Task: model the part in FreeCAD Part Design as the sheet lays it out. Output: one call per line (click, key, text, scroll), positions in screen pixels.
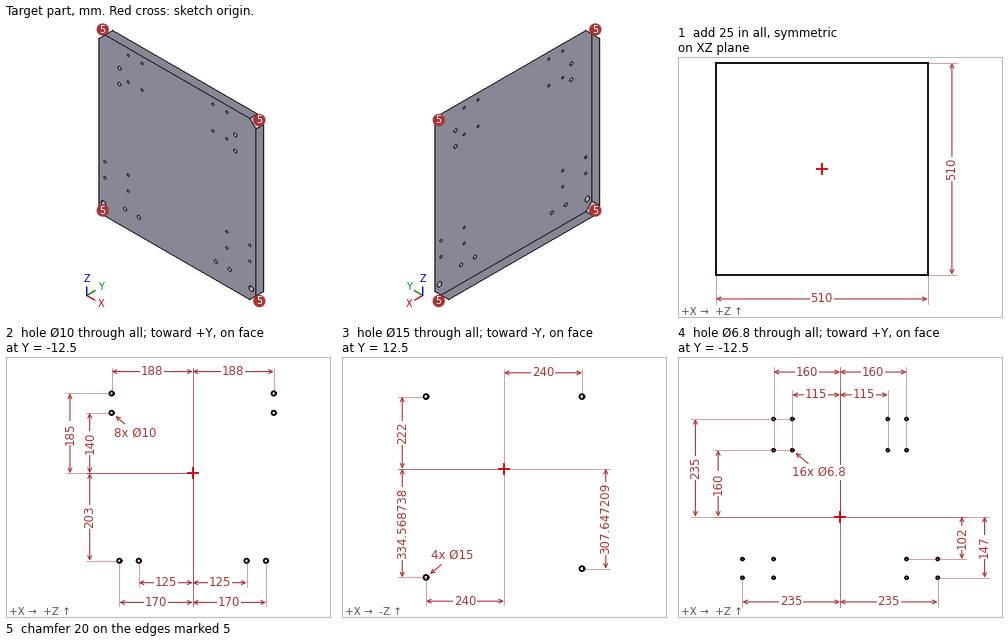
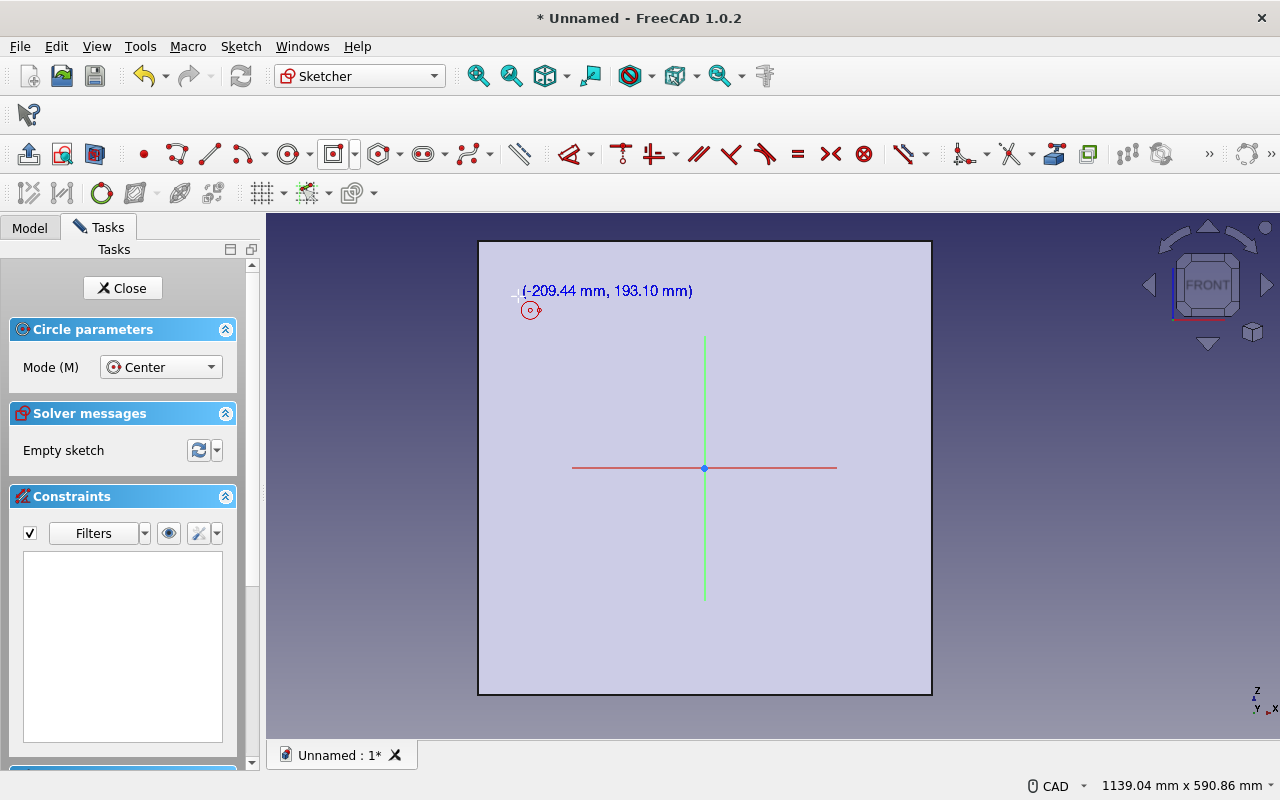
click(537, 304)
move(540, 300)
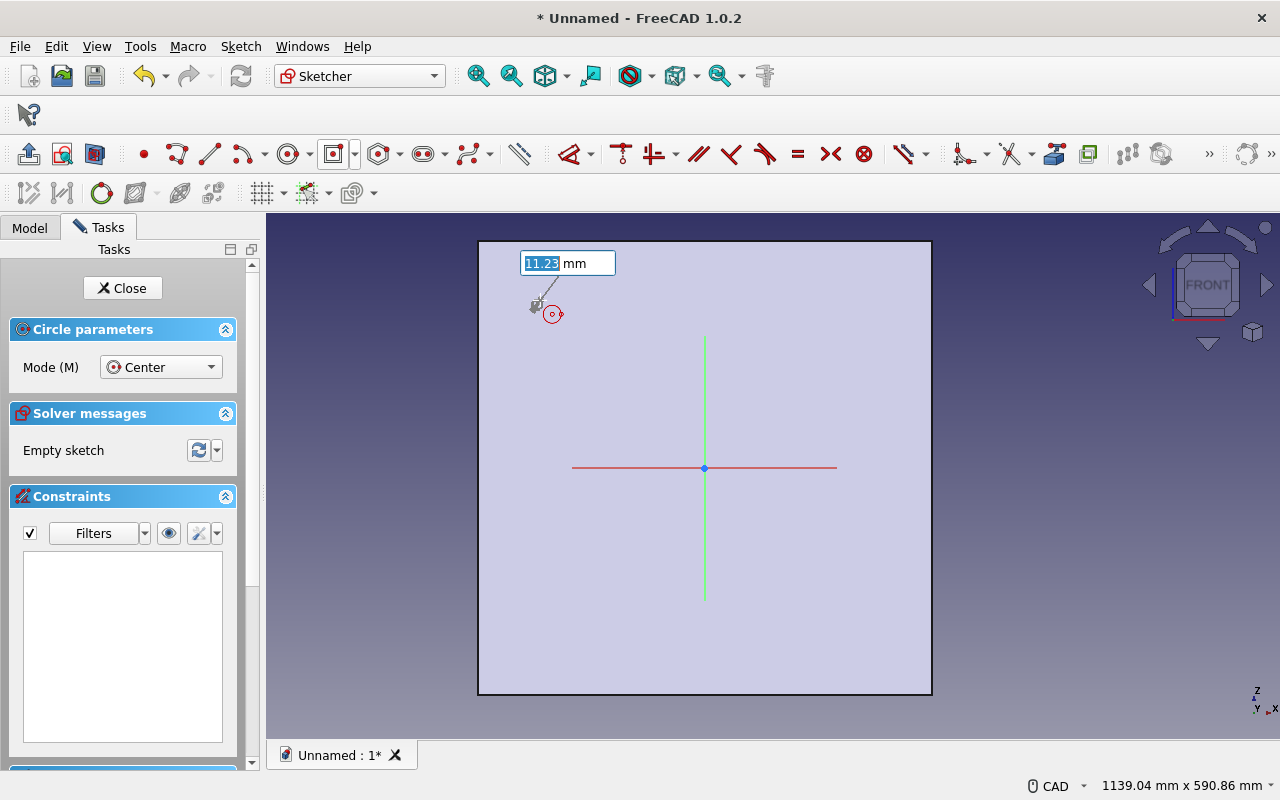
text(10)
key(Return)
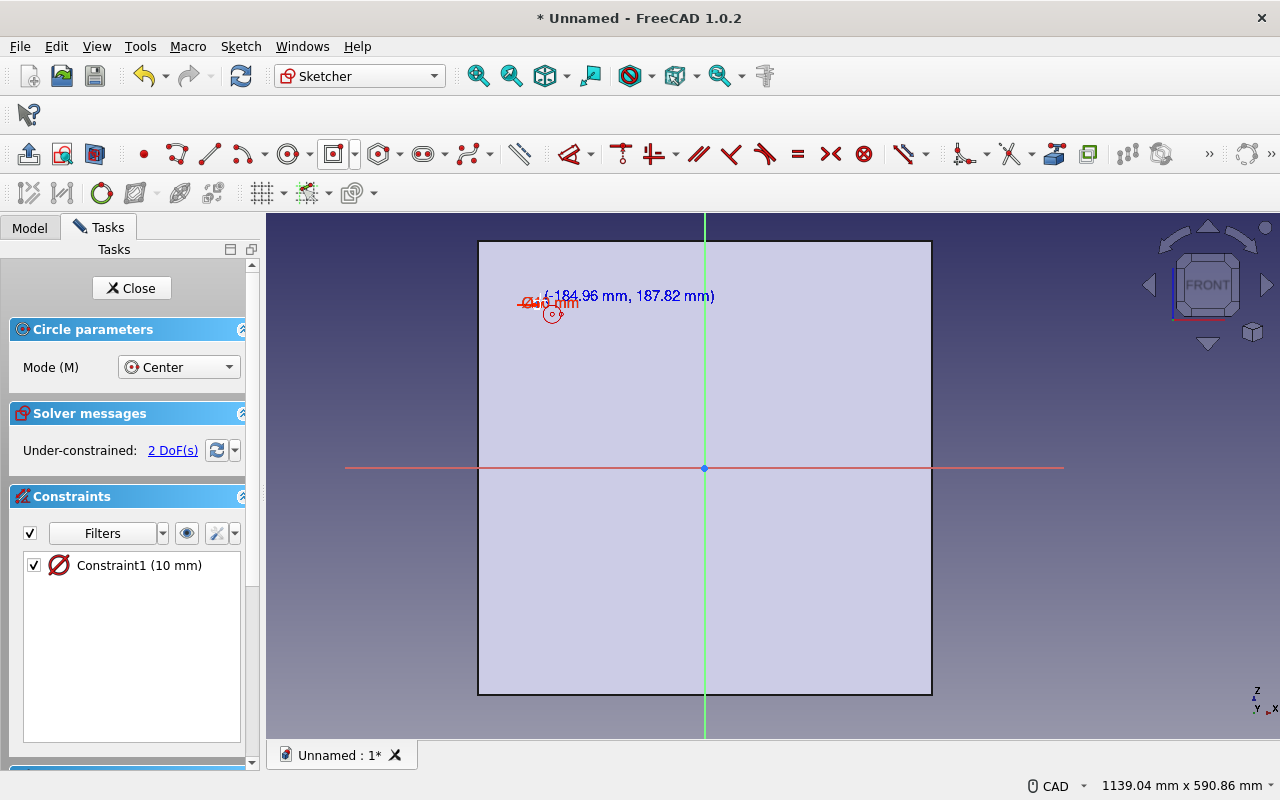
scroll(537, 344, up, 9)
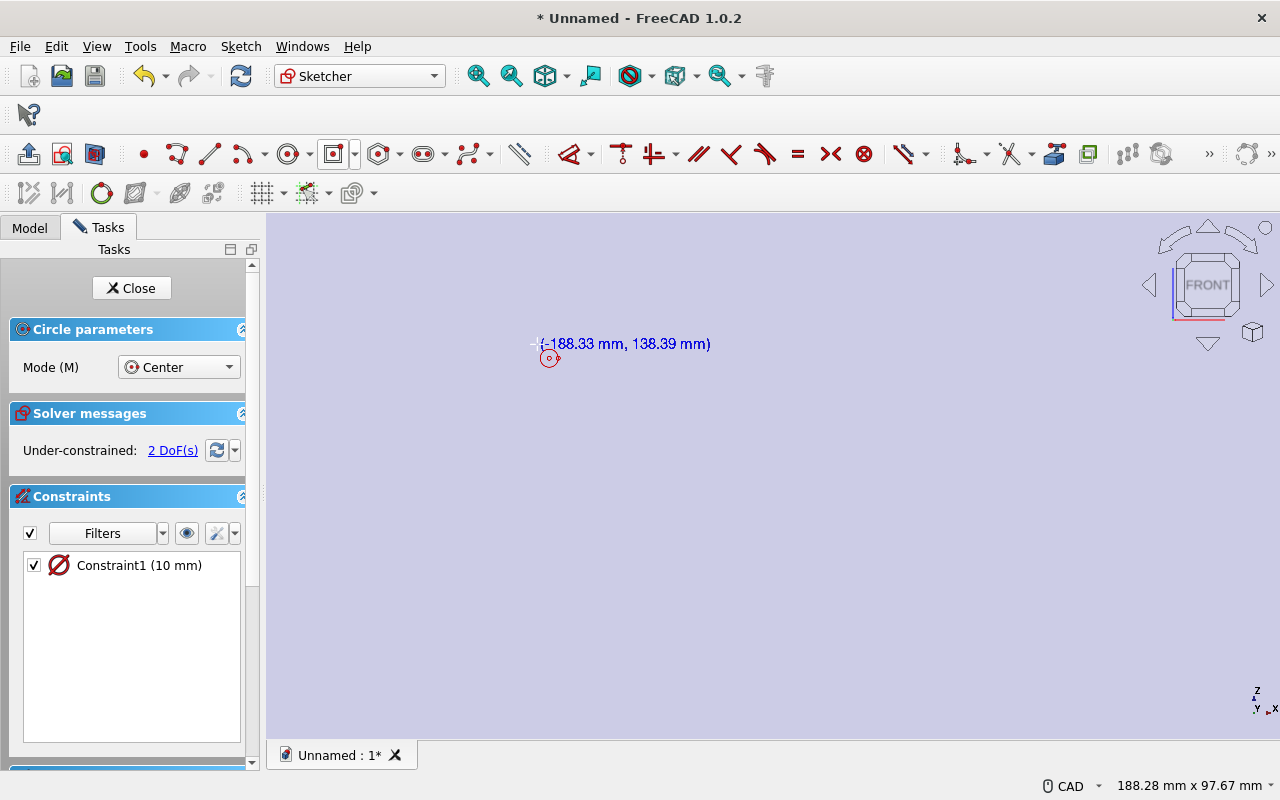
scroll(537, 344, down, 9)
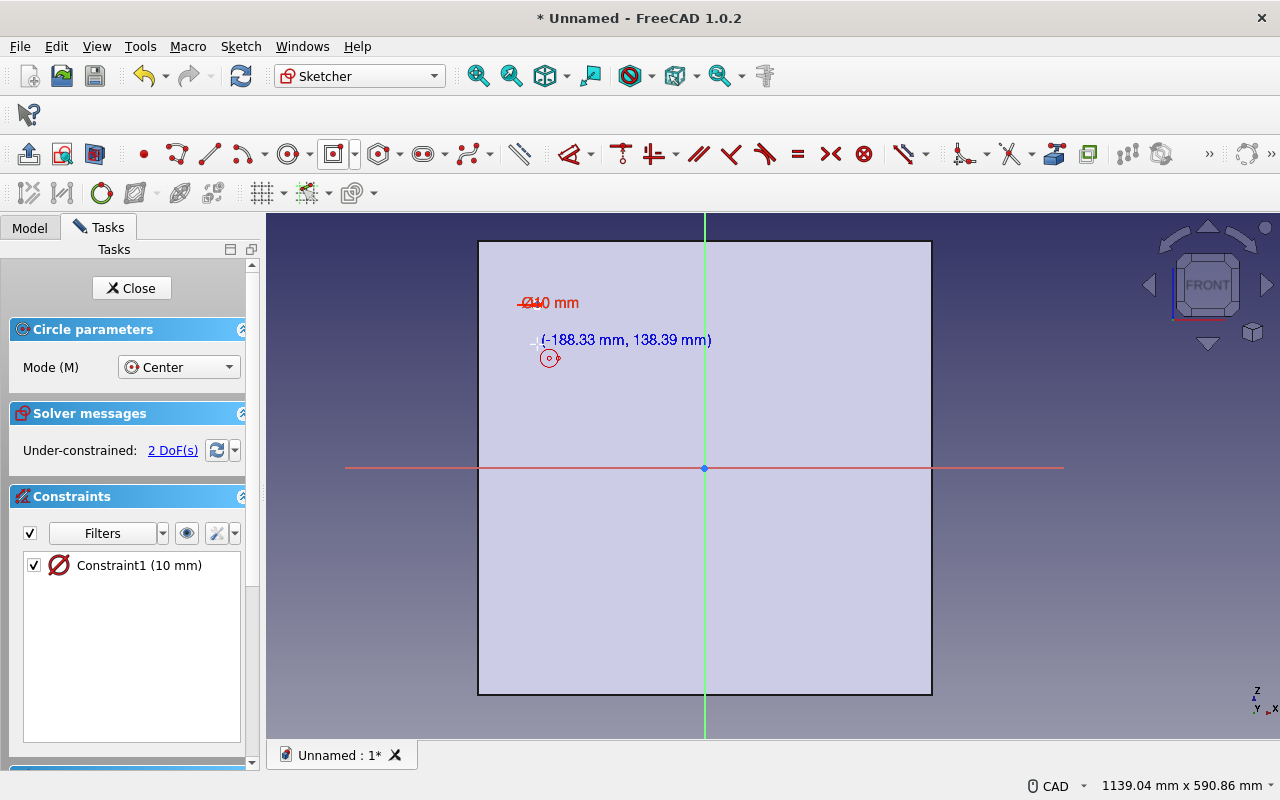
click(537, 344)
move(540, 340)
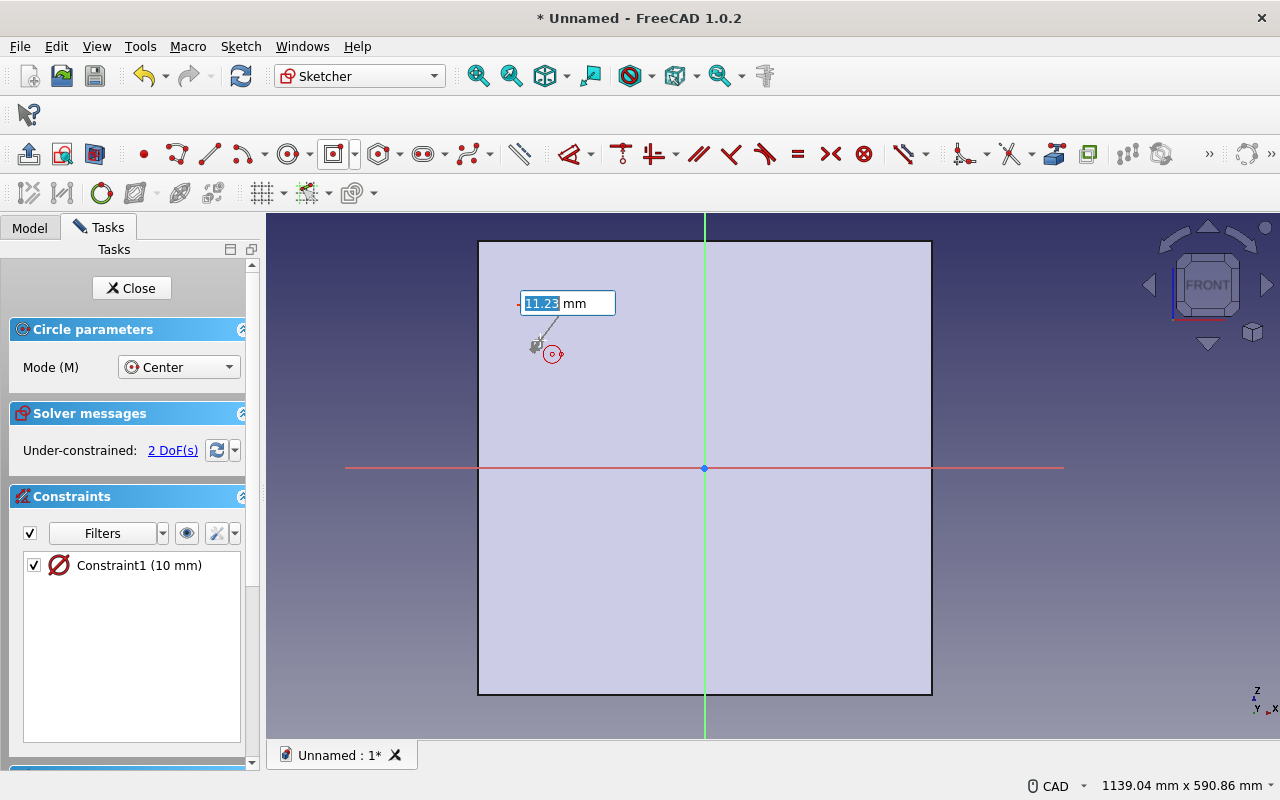
text(10)
key(Return)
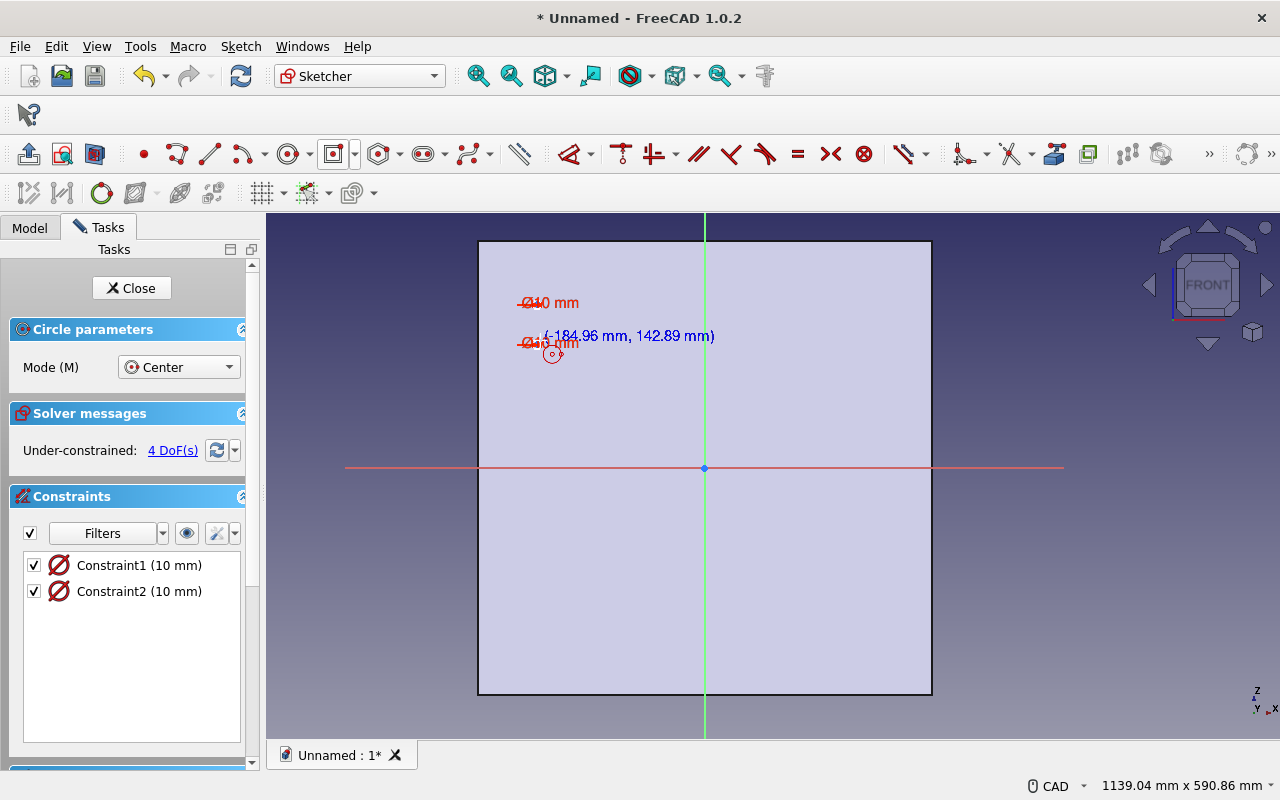
scroll(872, 304, up, 9)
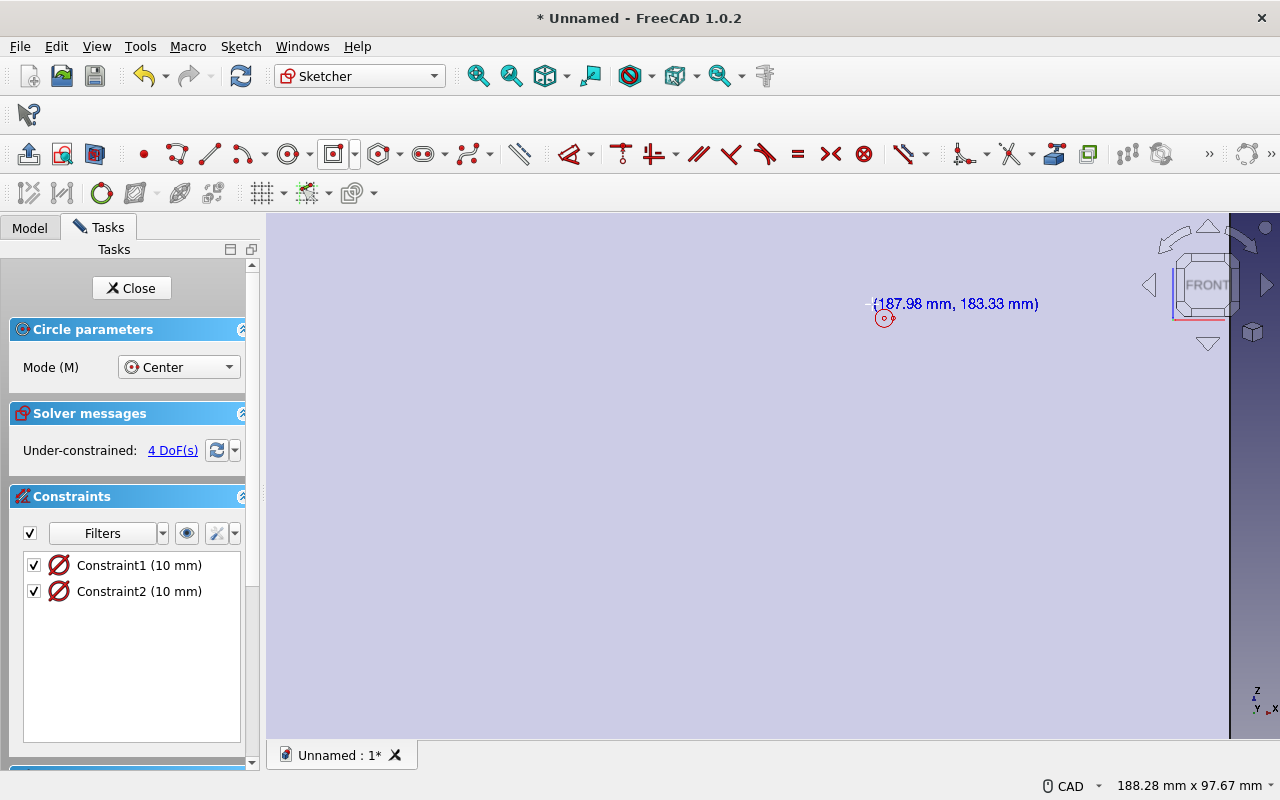
scroll(872, 304, down, 9)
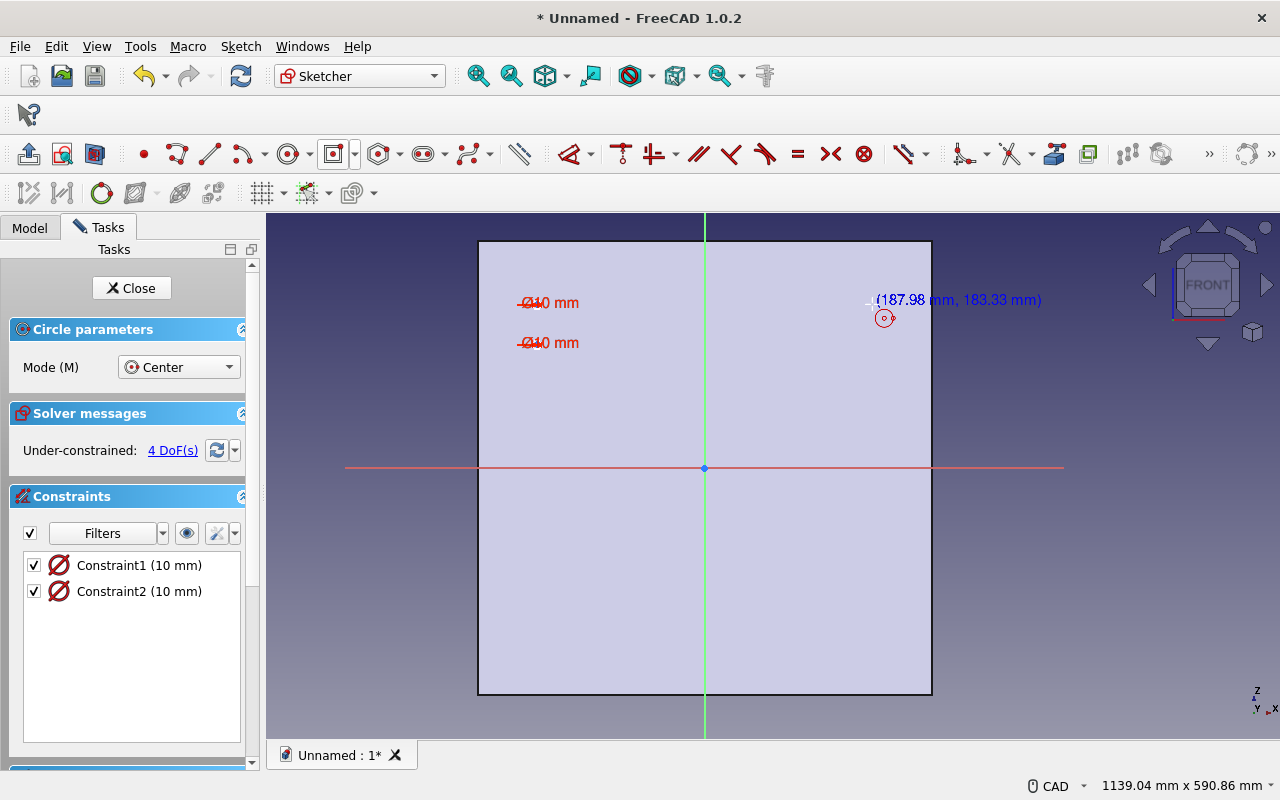
click(872, 304)
move(875, 300)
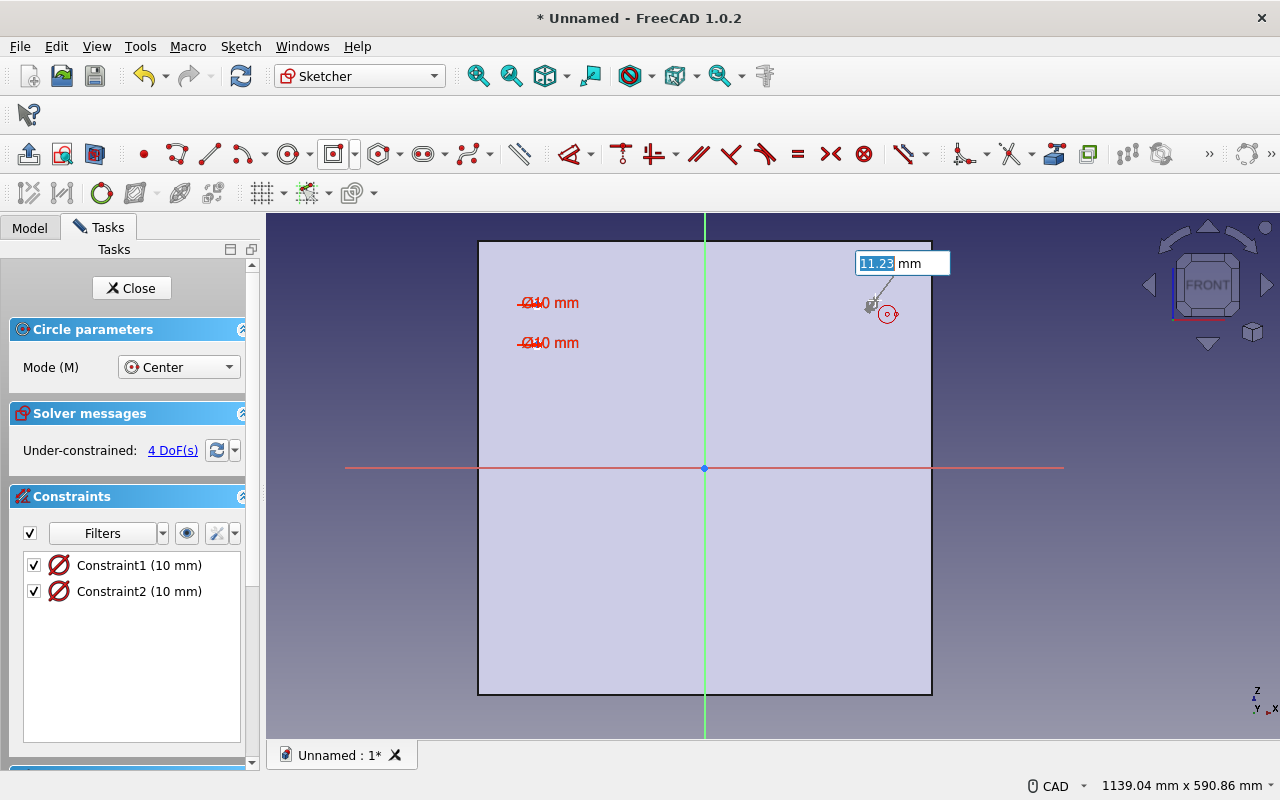
text(10)
key(Return)